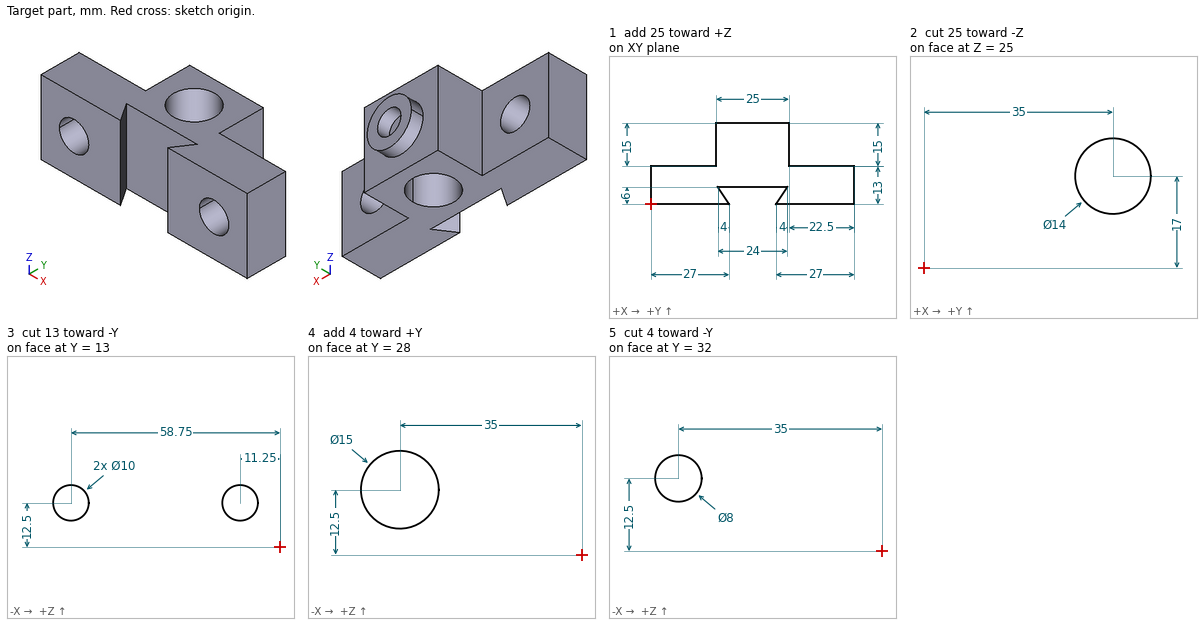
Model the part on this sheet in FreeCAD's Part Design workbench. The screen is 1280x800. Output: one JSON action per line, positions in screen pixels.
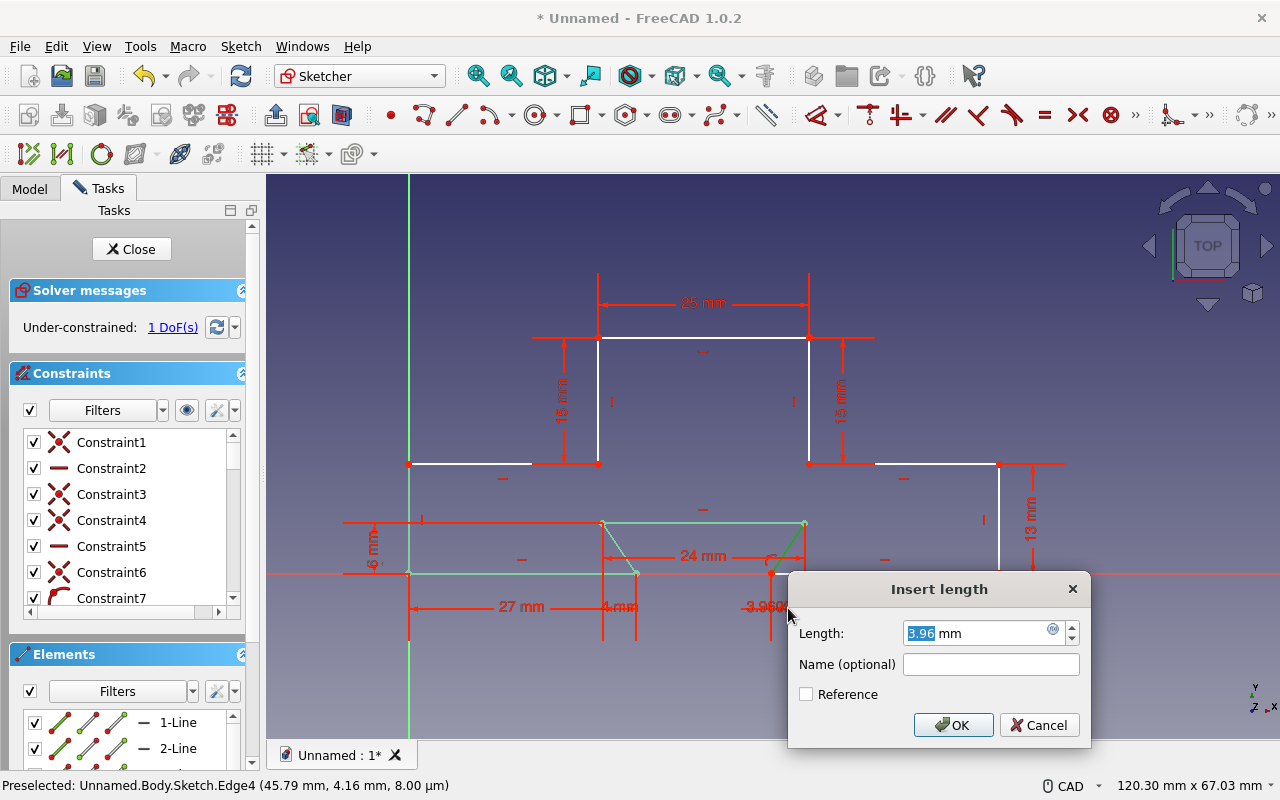
{"action": "type", "text": "4"}
{"action": "key", "text": "Return"}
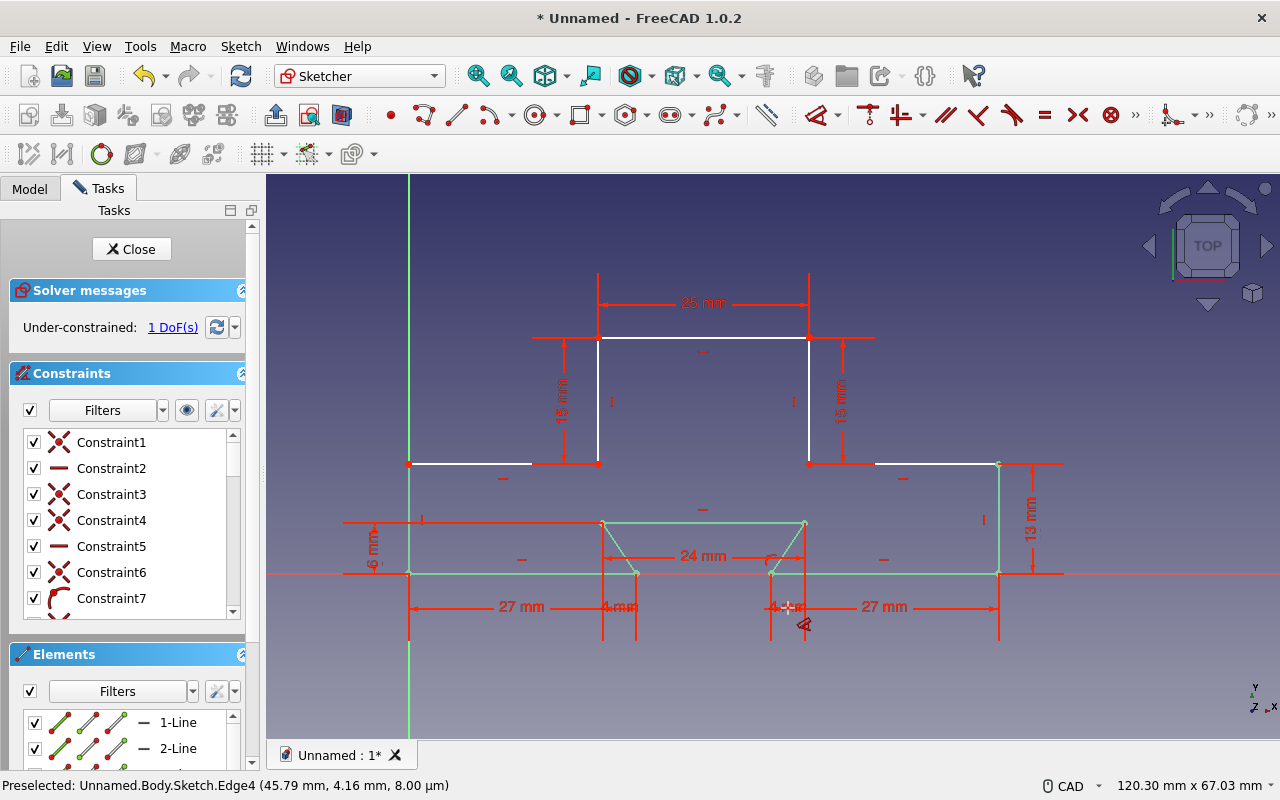
{"action": "left_click", "coordinate": [942, 464]}
{"action": "left_click", "coordinate": [904, 498]}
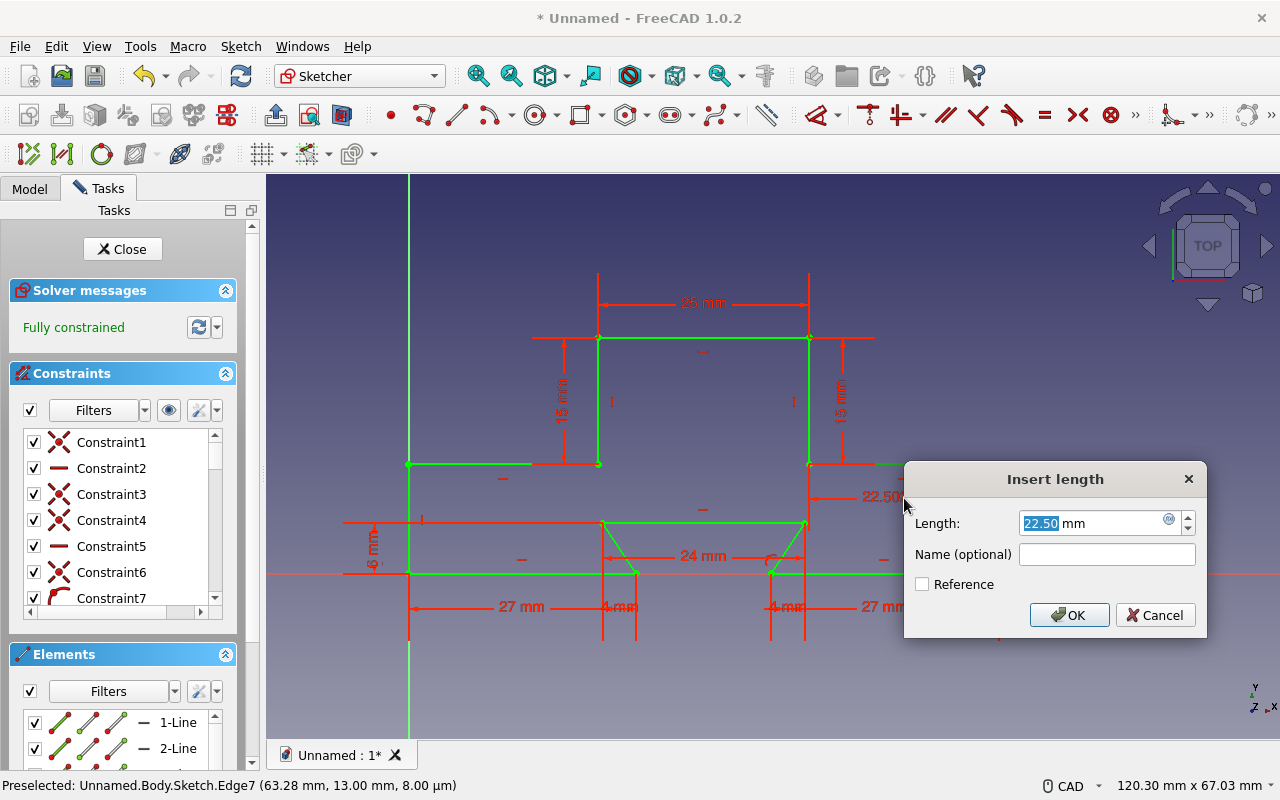
{"action": "type", "text": "22.5"}
{"action": "key", "text": "Return"}
{"action": "key", "text": "Escape"}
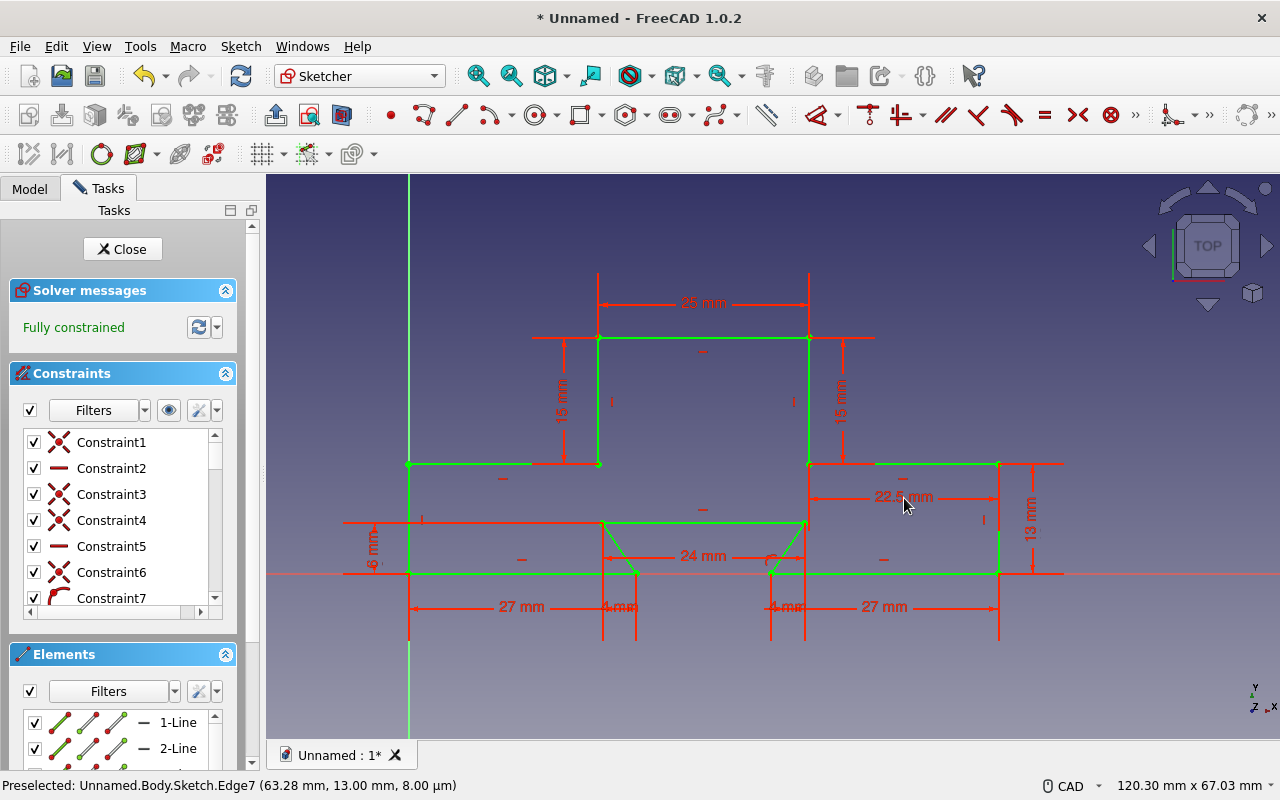
{"action": "left_click", "coordinate": [123, 249]}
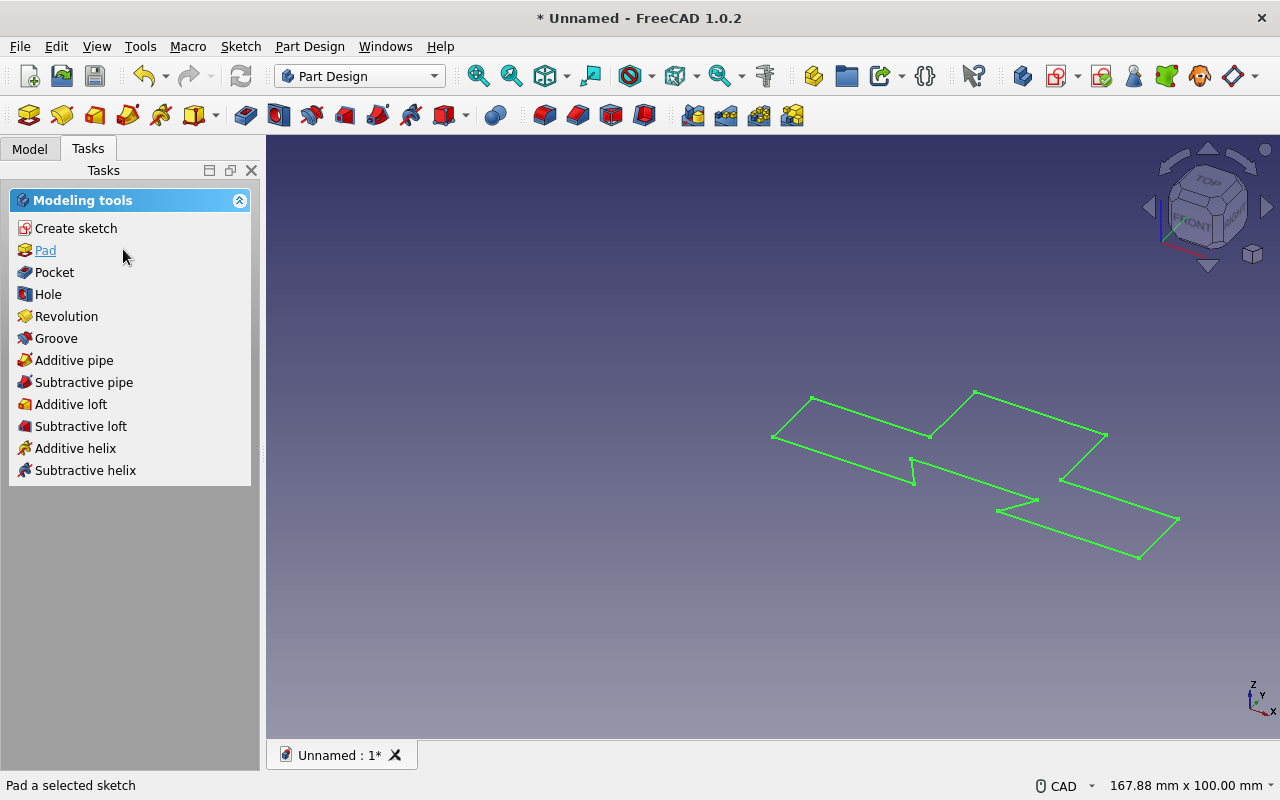
{"action": "left_click", "coordinate": [29, 116]}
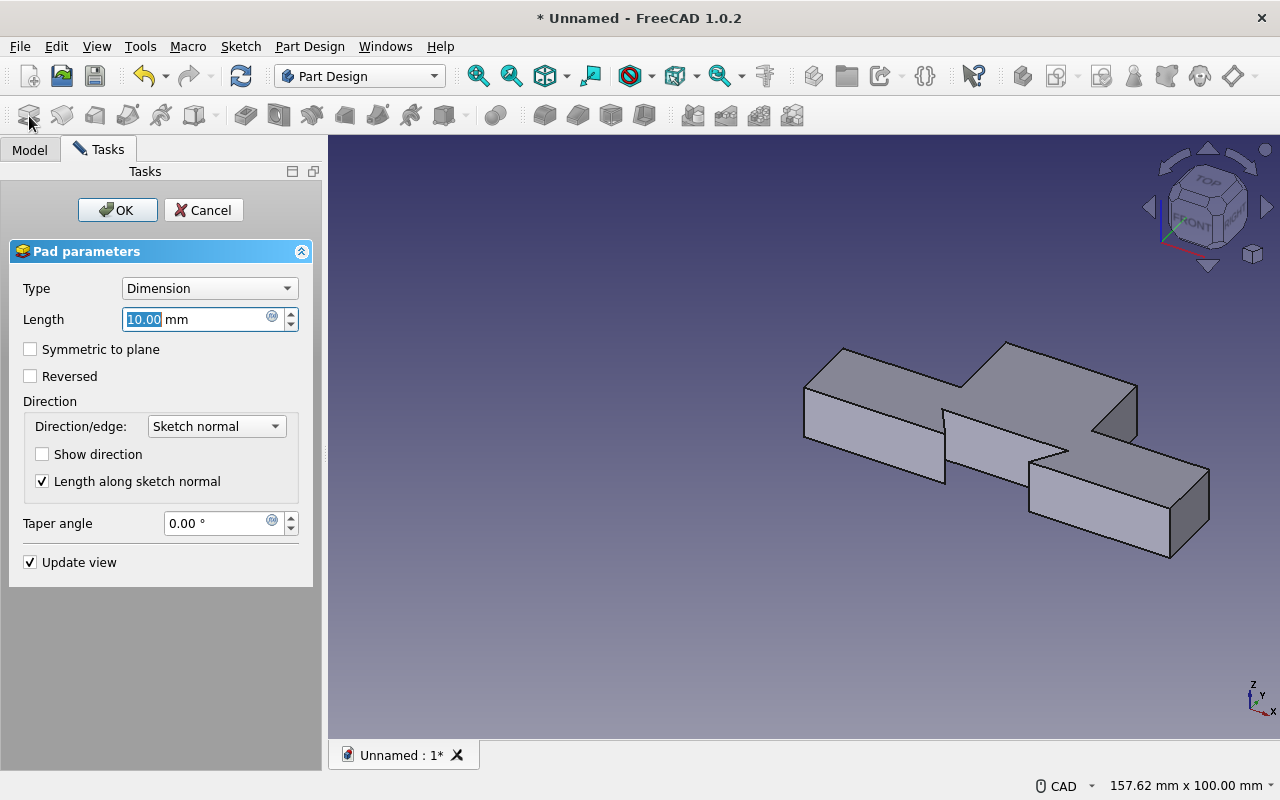
{"action": "type", "text": "25"}
{"action": "key", "text": "Tab"}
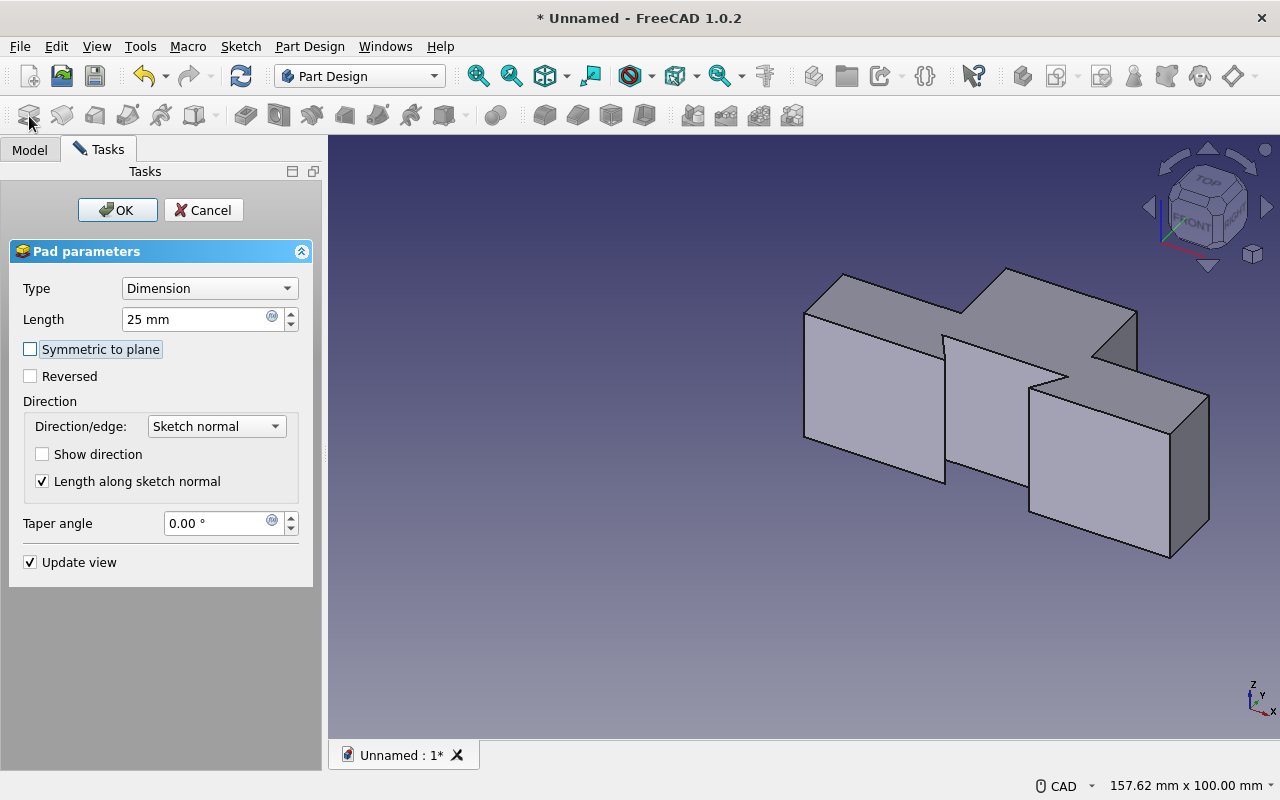
{"action": "left_click", "coordinate": [118, 210]}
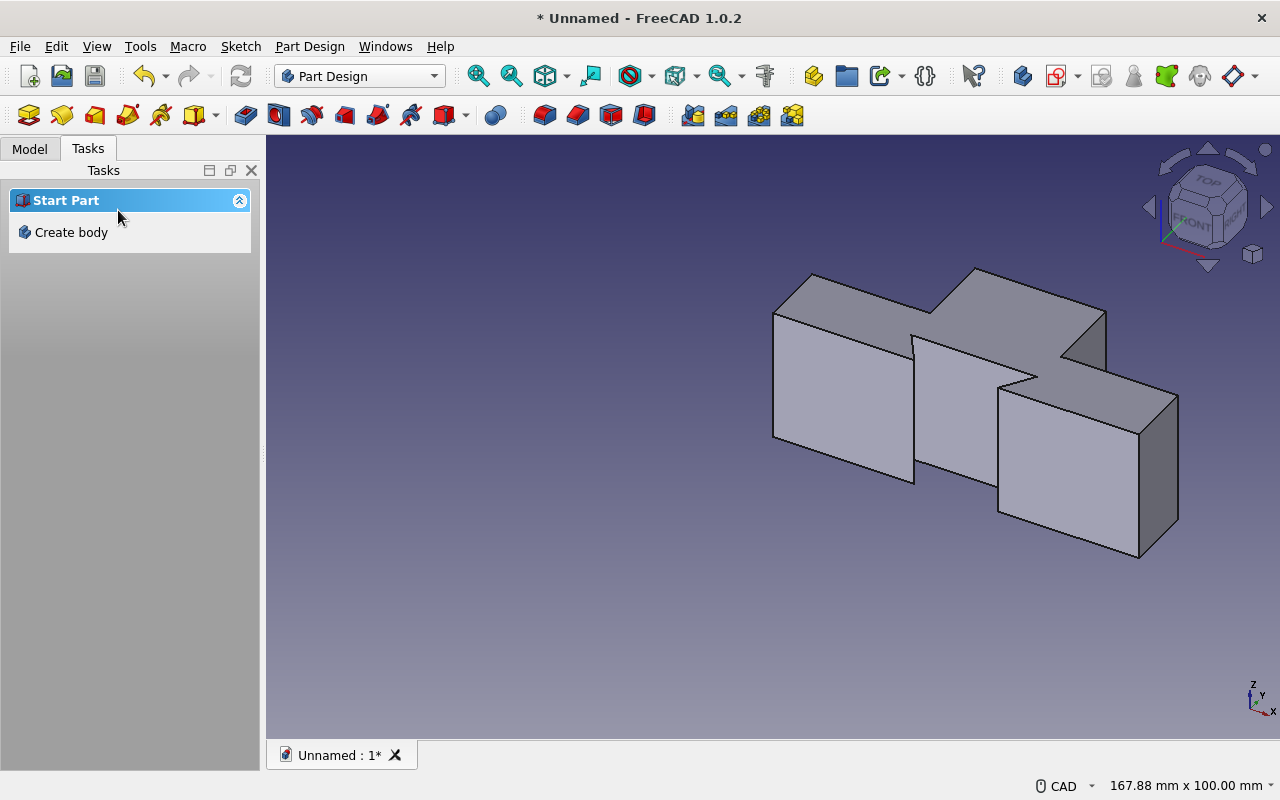
{"action": "left_click", "coordinate": [1010, 319]}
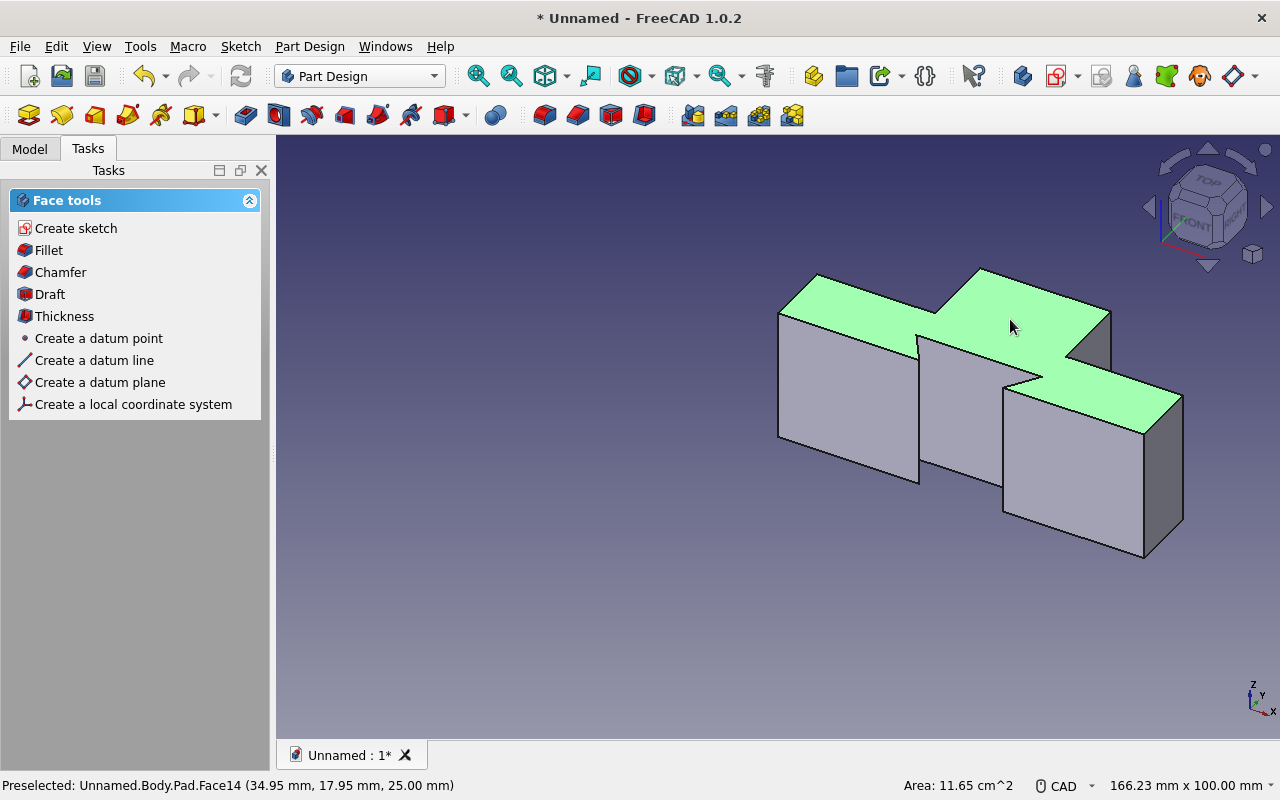
{"action": "left_click", "coordinate": [1056, 76]}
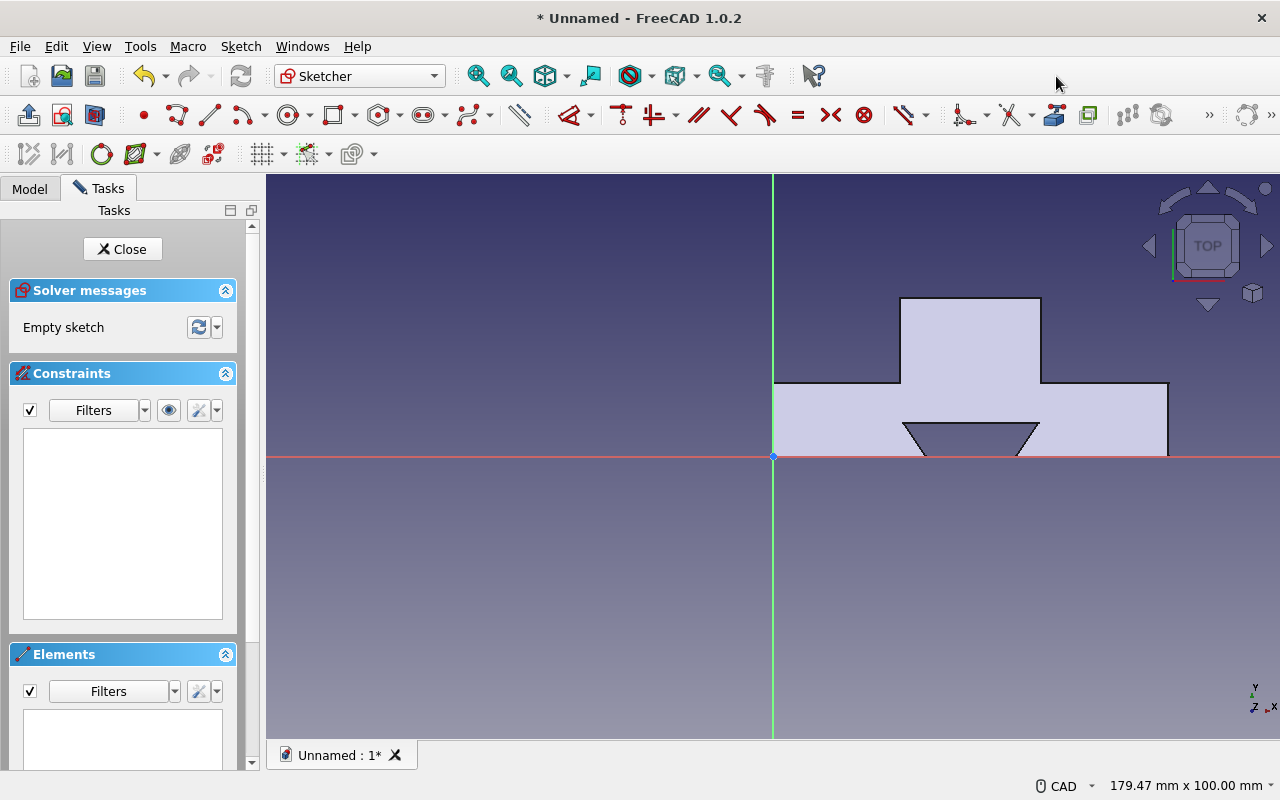
{"action": "scroll", "coordinate": [1038, 336], "scroll_direction": "up", "scroll_amount": 8}